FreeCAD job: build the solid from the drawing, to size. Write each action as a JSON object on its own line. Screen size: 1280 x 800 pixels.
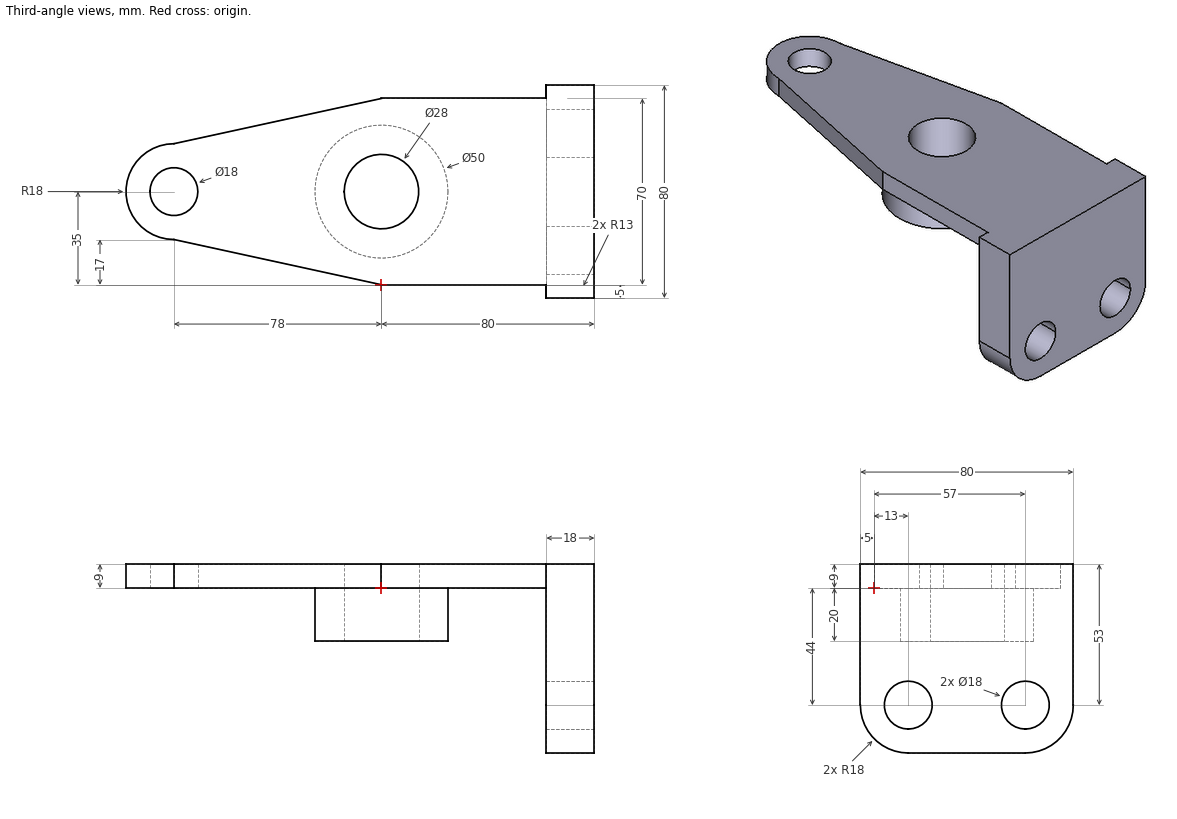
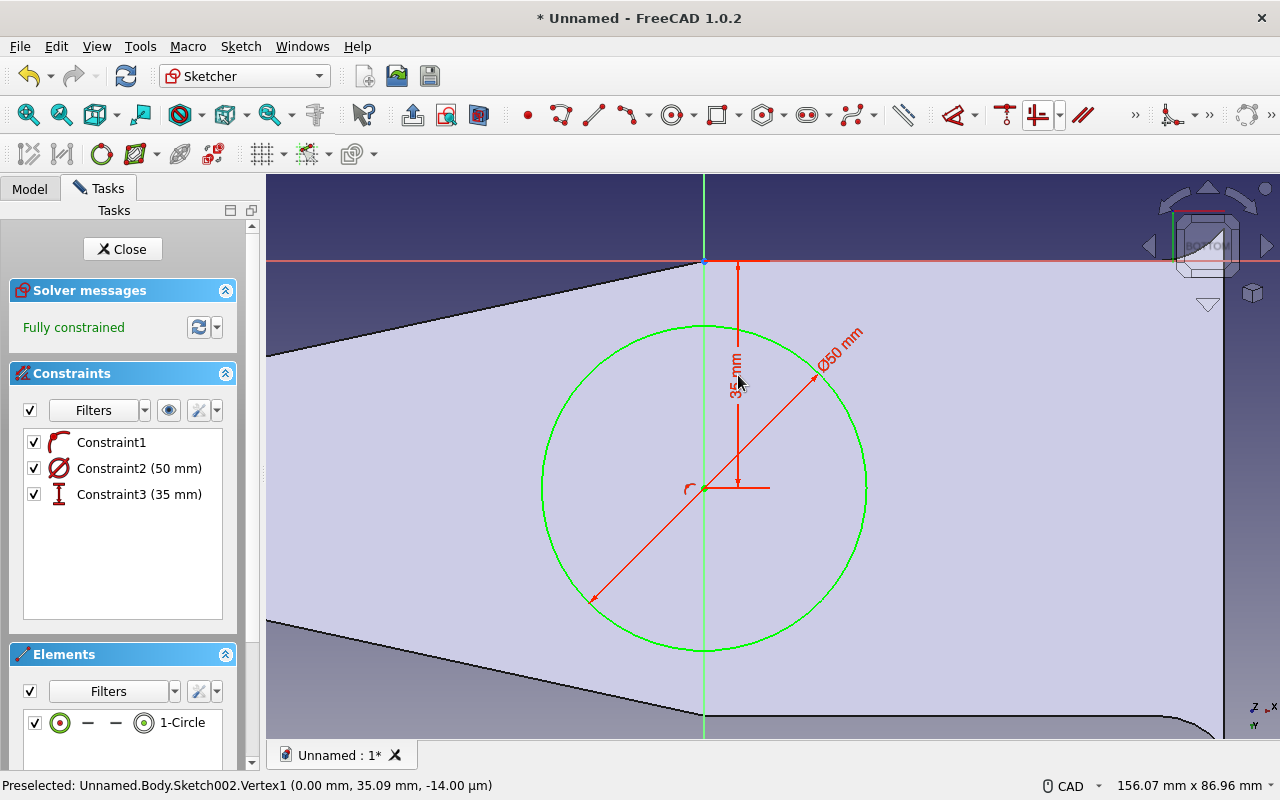
{"action": "left_click", "coordinate": [123, 249]}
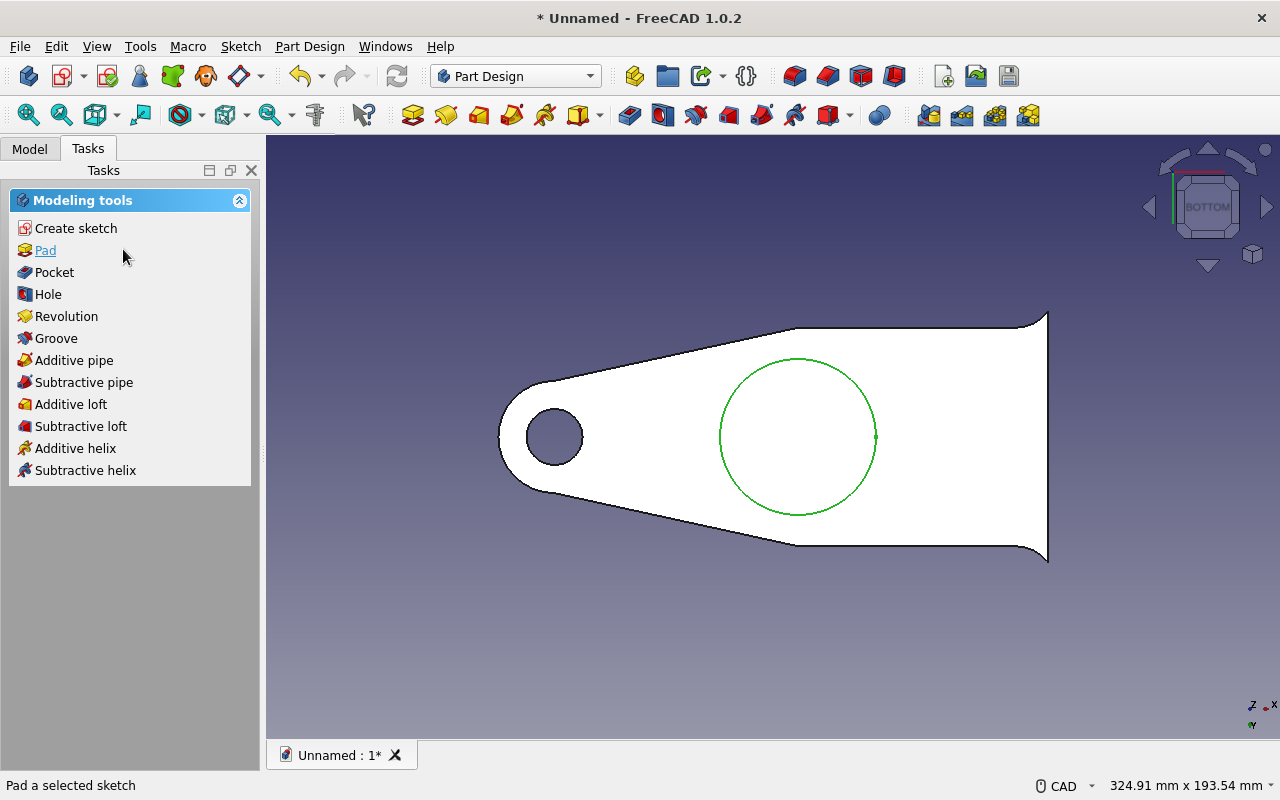
{"action": "left_click", "coordinate": [413, 116]}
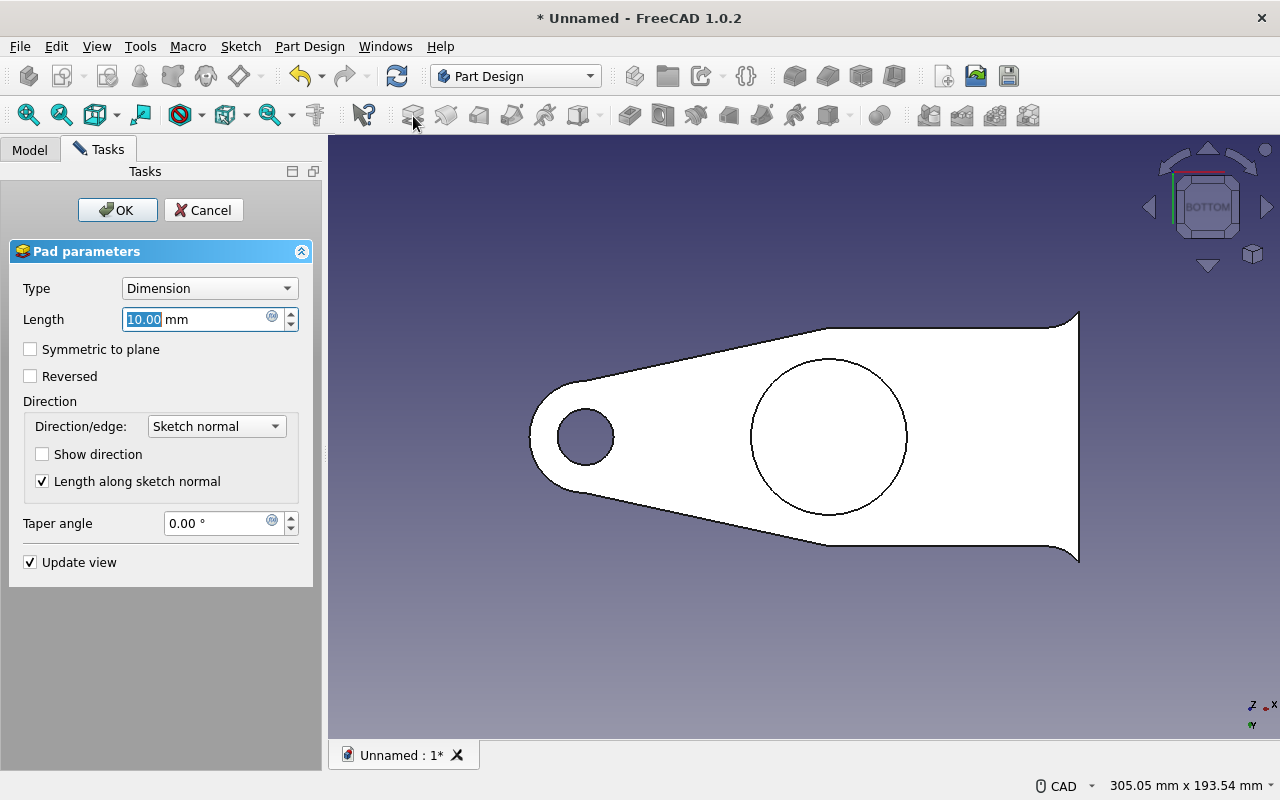
{"action": "type", "text": "20"}
{"action": "key", "text": "Tab"}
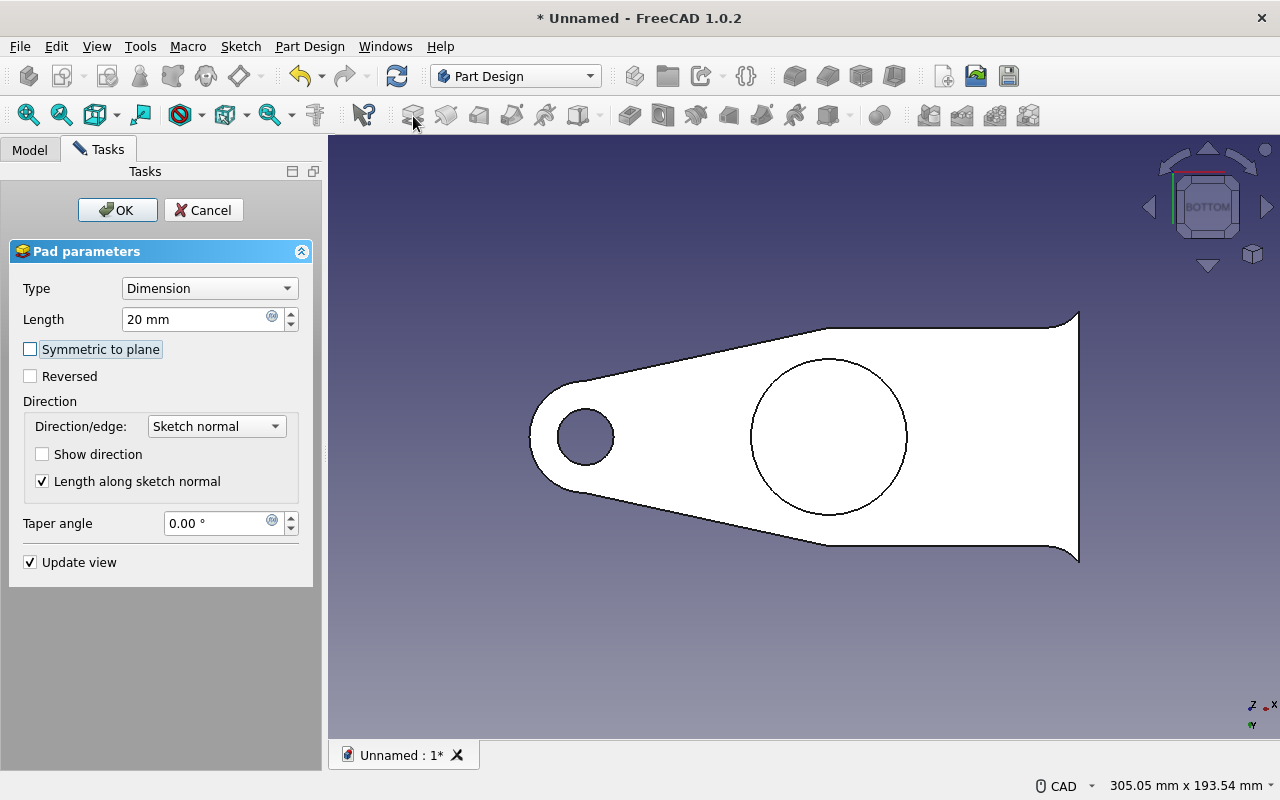
{"action": "left_click", "coordinate": [118, 210]}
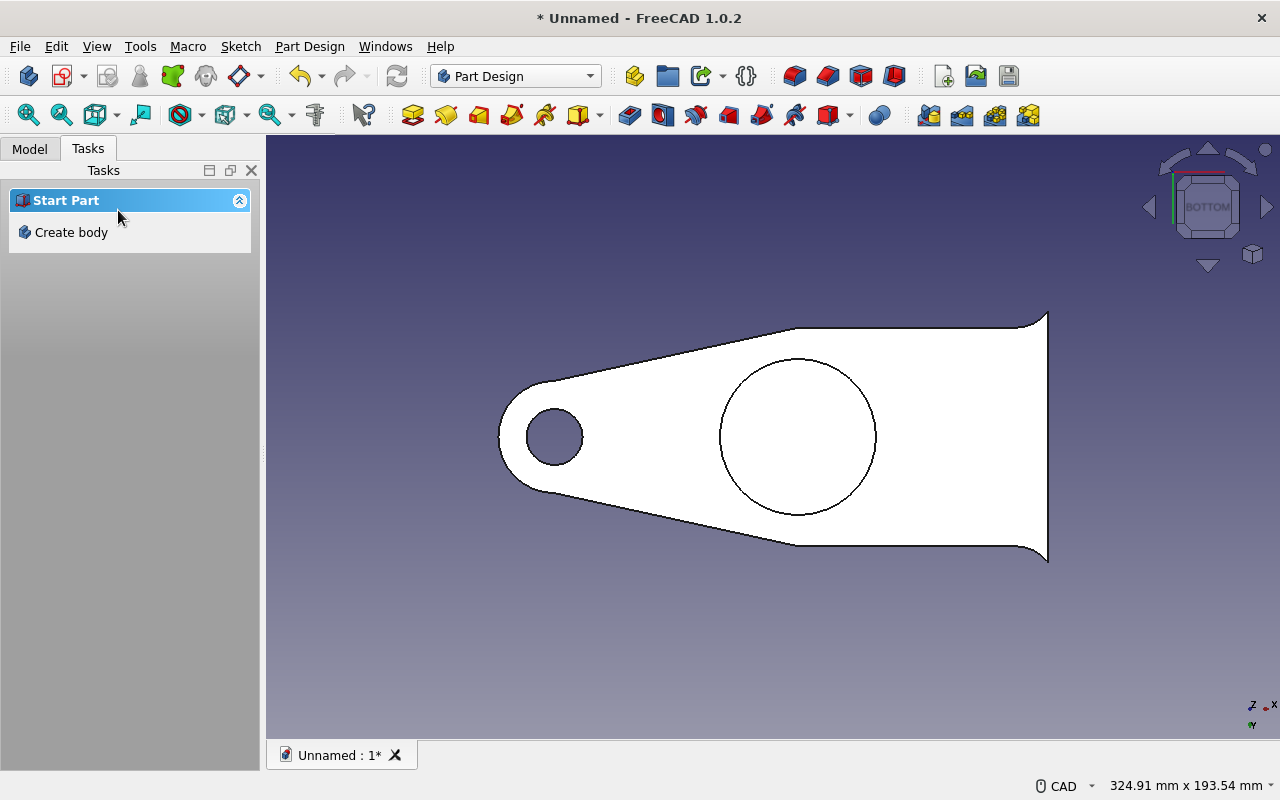
{"action": "left_click", "coordinate": [798, 436]}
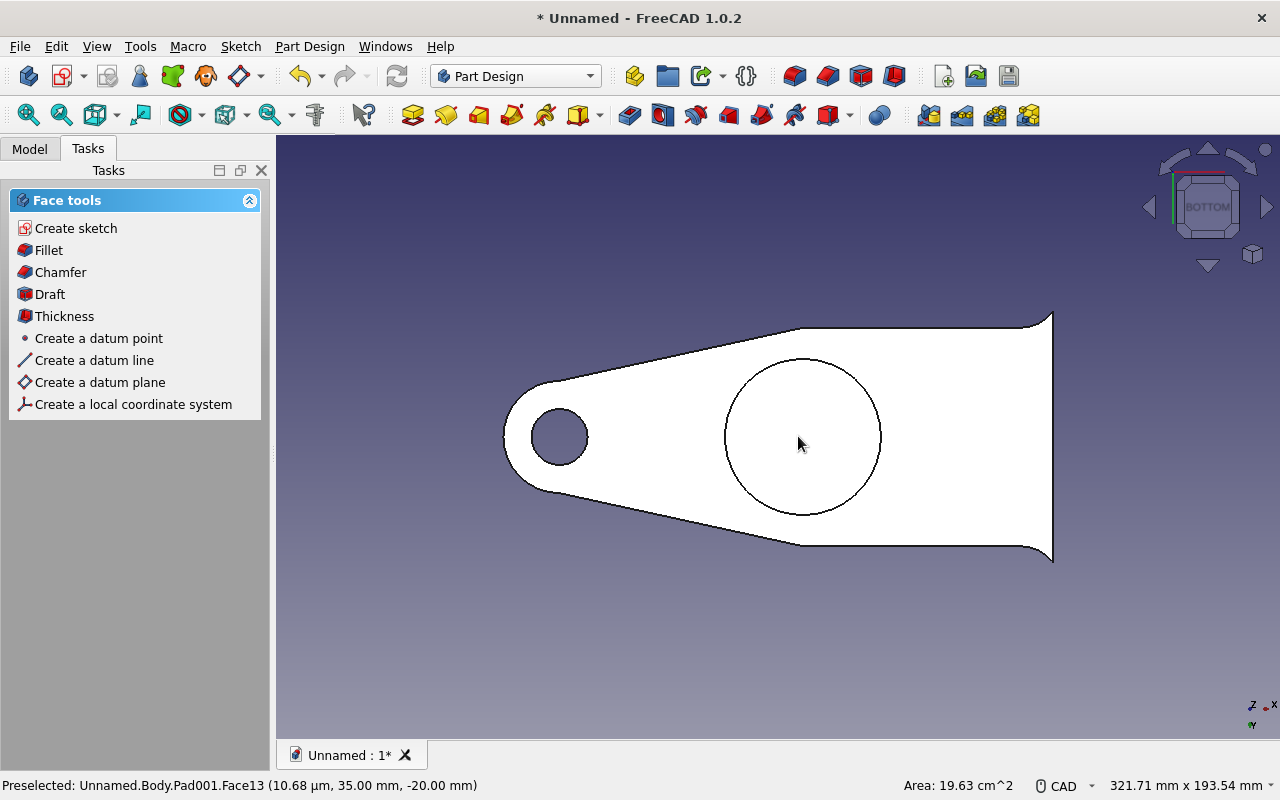
{"action": "left_click", "coordinate": [62, 76]}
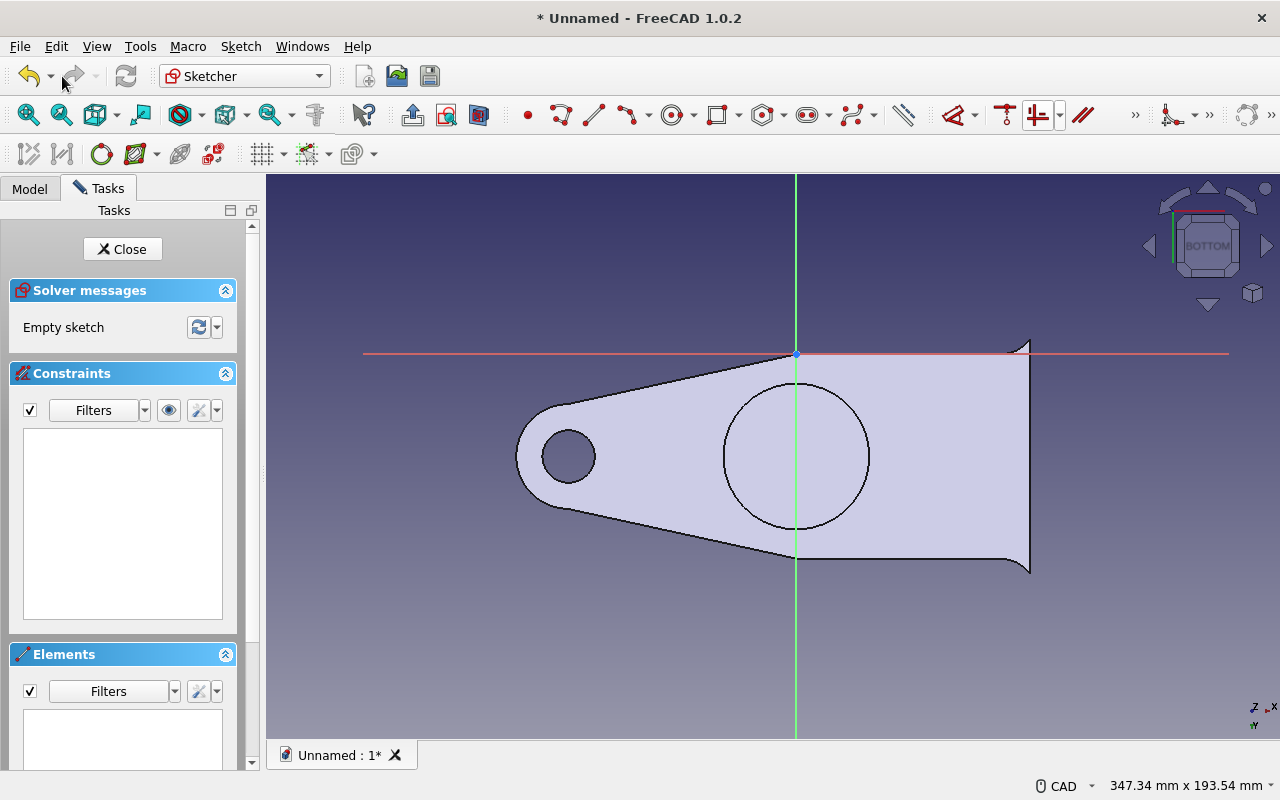
{"action": "scroll", "coordinate": [850, 408], "scroll_direction": "up", "scroll_amount": 5}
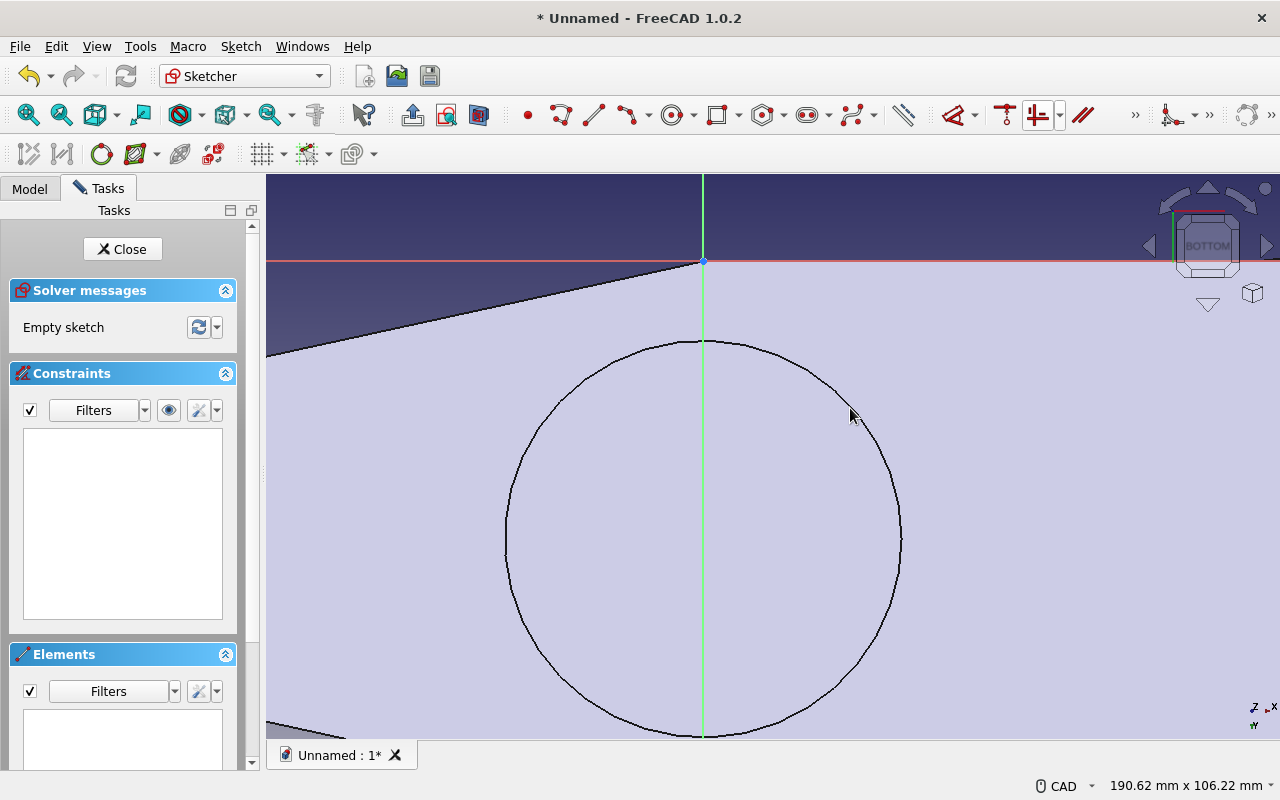
{"action": "left_click", "coordinate": [672, 116]}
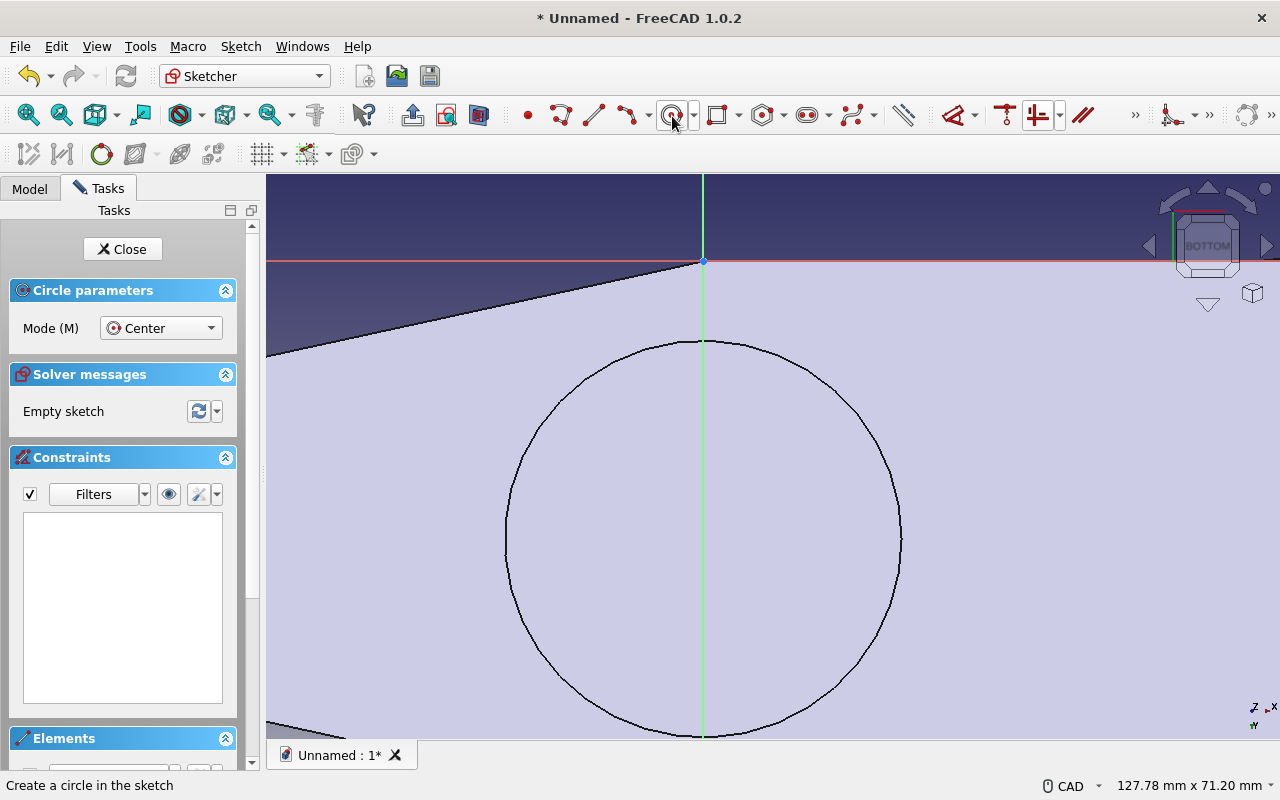
{"action": "left_click", "coordinate": [703, 539]}
{"action": "left_click", "coordinate": [782, 461]}
{"action": "key", "text": "Escape"}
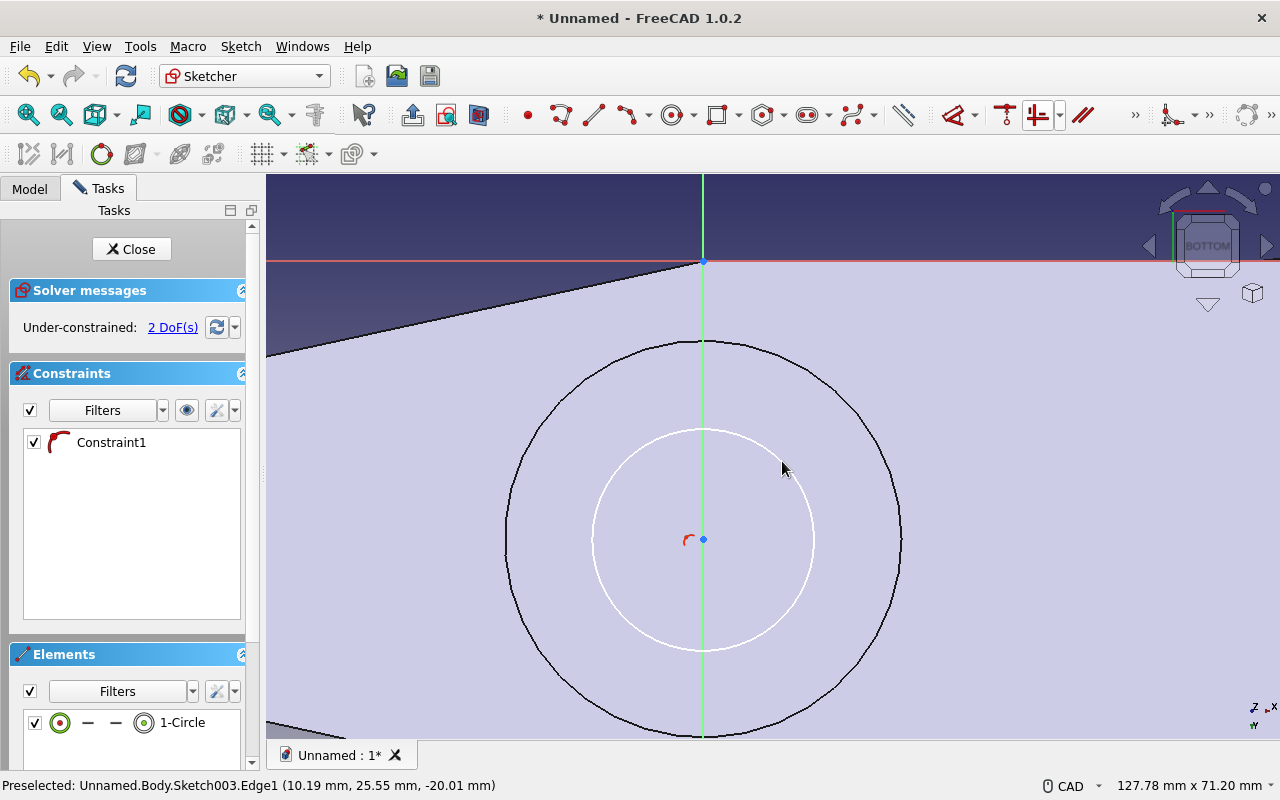
{"action": "key", "text": "d"}